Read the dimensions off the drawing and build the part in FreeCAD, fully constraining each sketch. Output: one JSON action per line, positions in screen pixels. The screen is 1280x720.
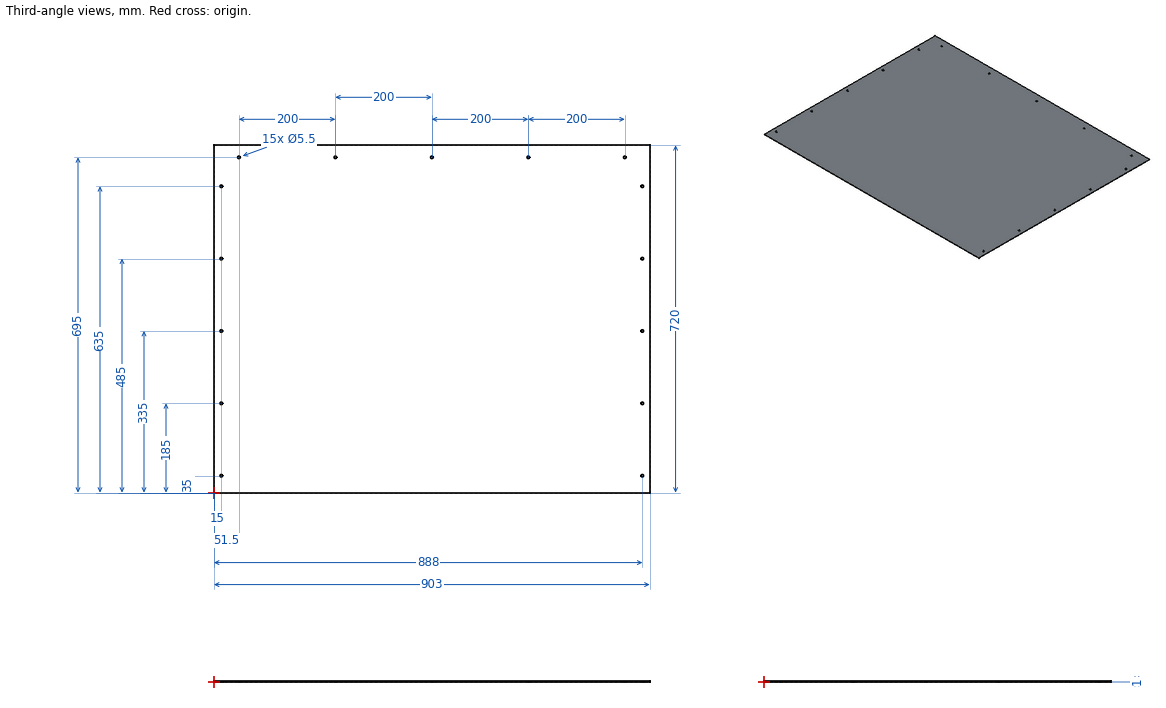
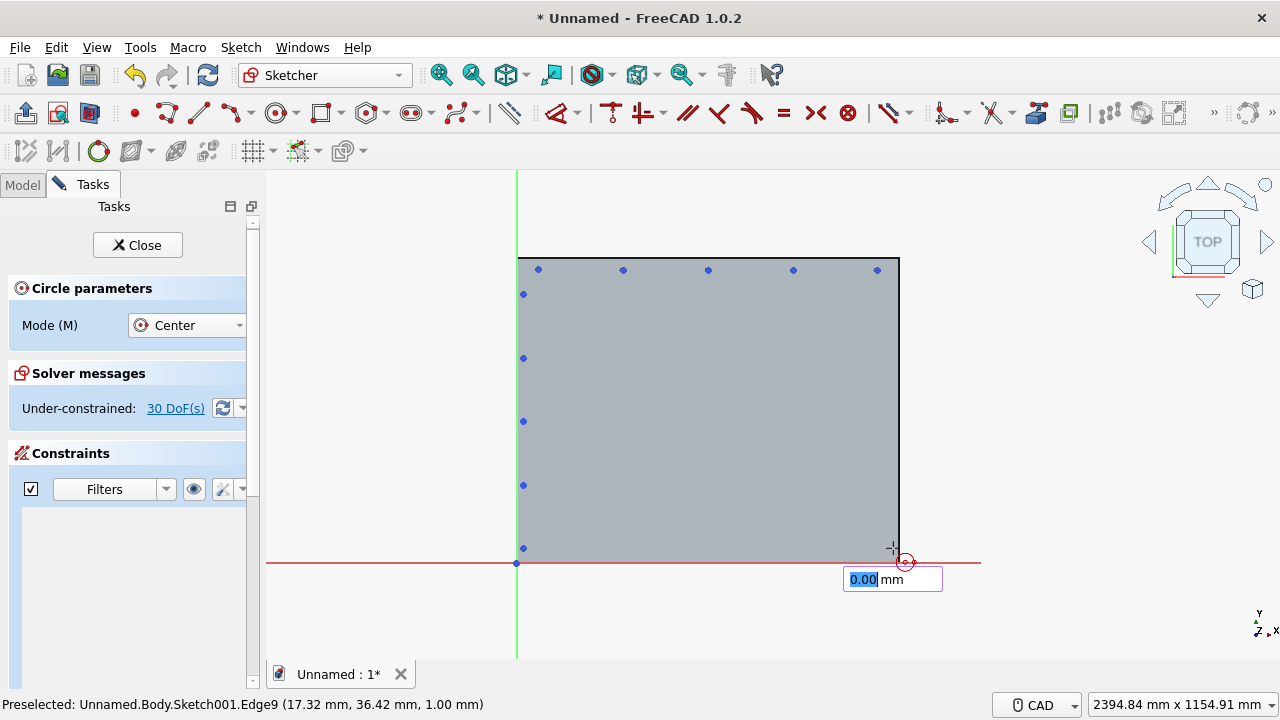
{"action": "scroll", "coordinate": [894, 547], "scroll_direction": "up", "scroll_amount": 14}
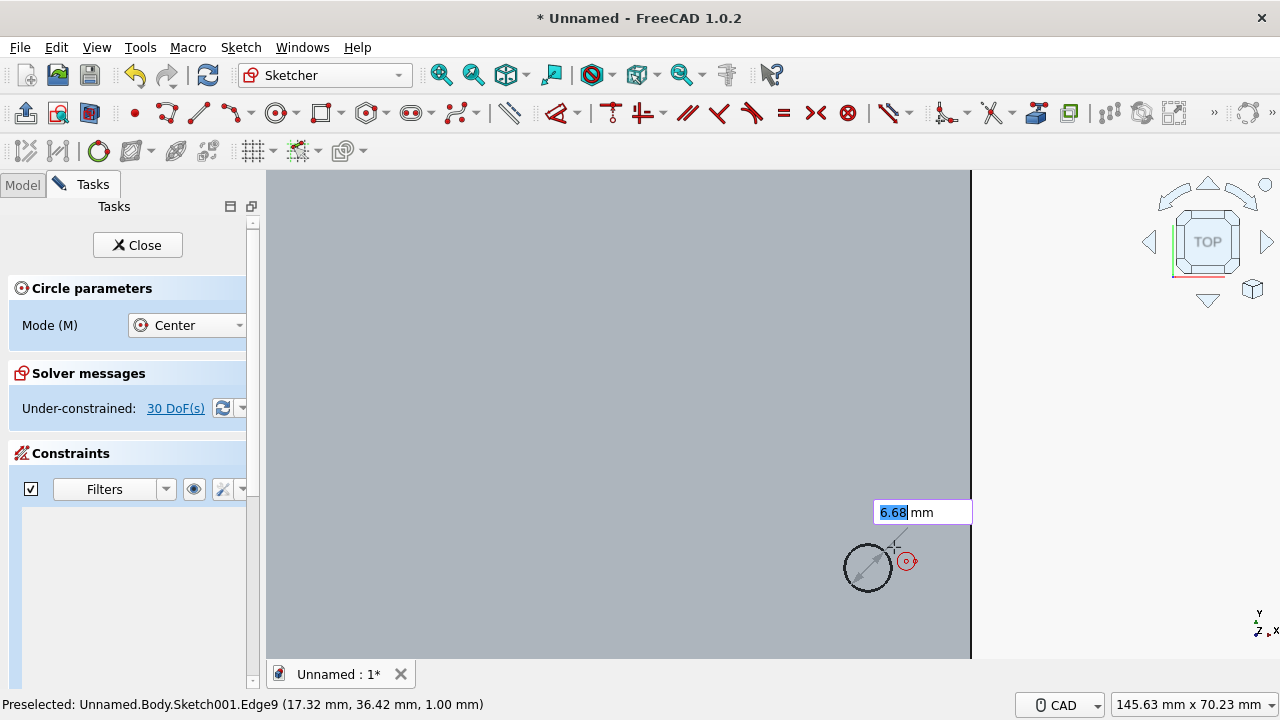
{"action": "left_click", "coordinate": [880, 541]}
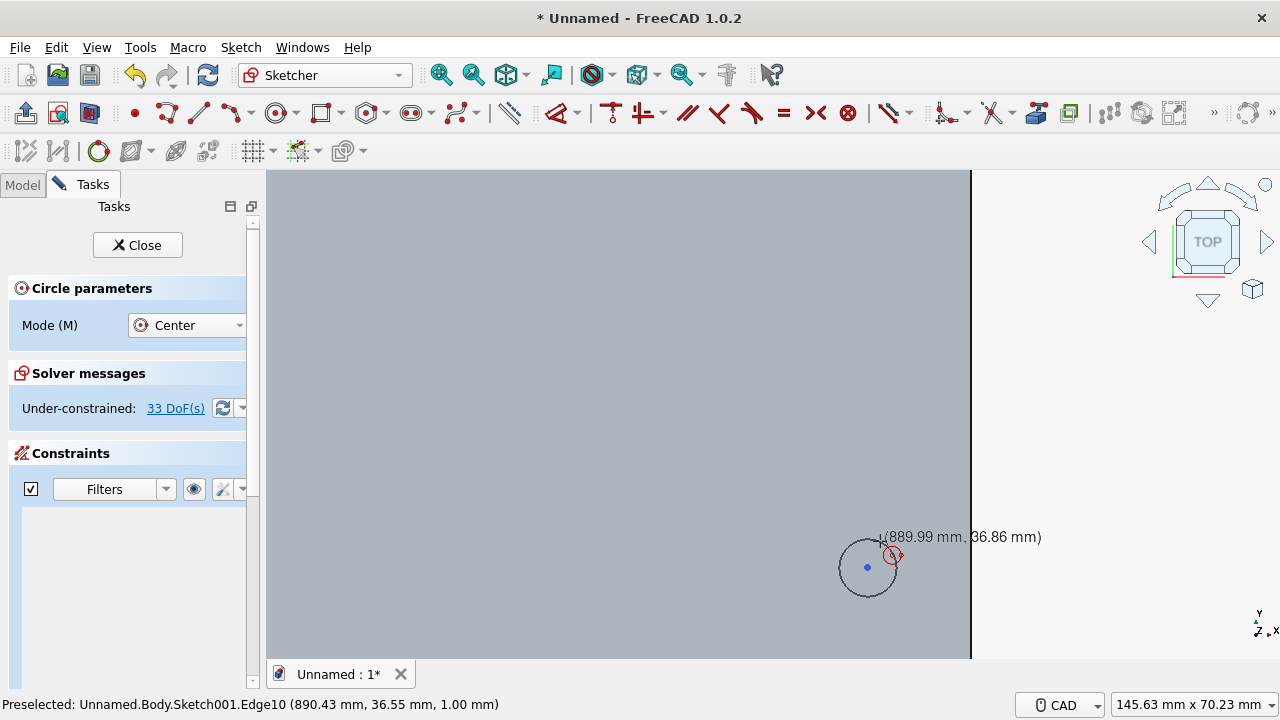
{"action": "scroll", "coordinate": [894, 547], "scroll_direction": "down", "scroll_amount": 14}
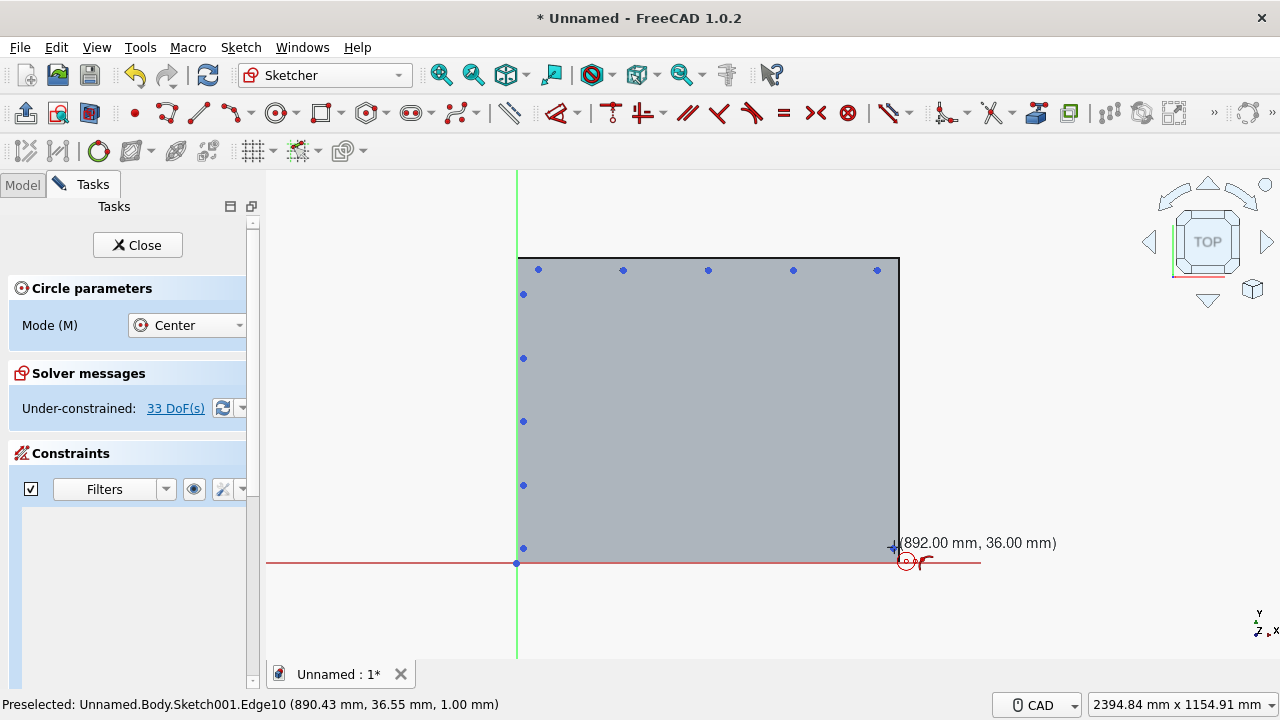
{"action": "scroll", "coordinate": [893, 485], "scroll_direction": "up", "scroll_amount": 15}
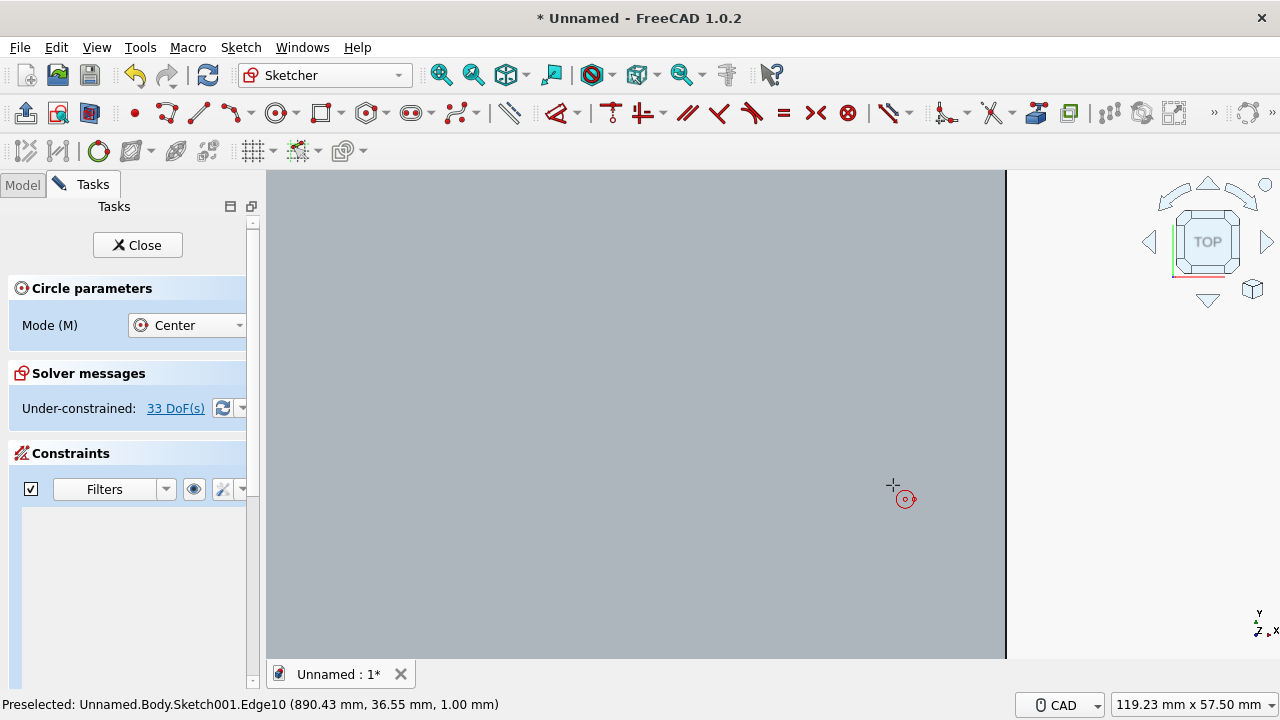
{"action": "scroll", "coordinate": [893, 485], "scroll_direction": "down", "scroll_amount": 15}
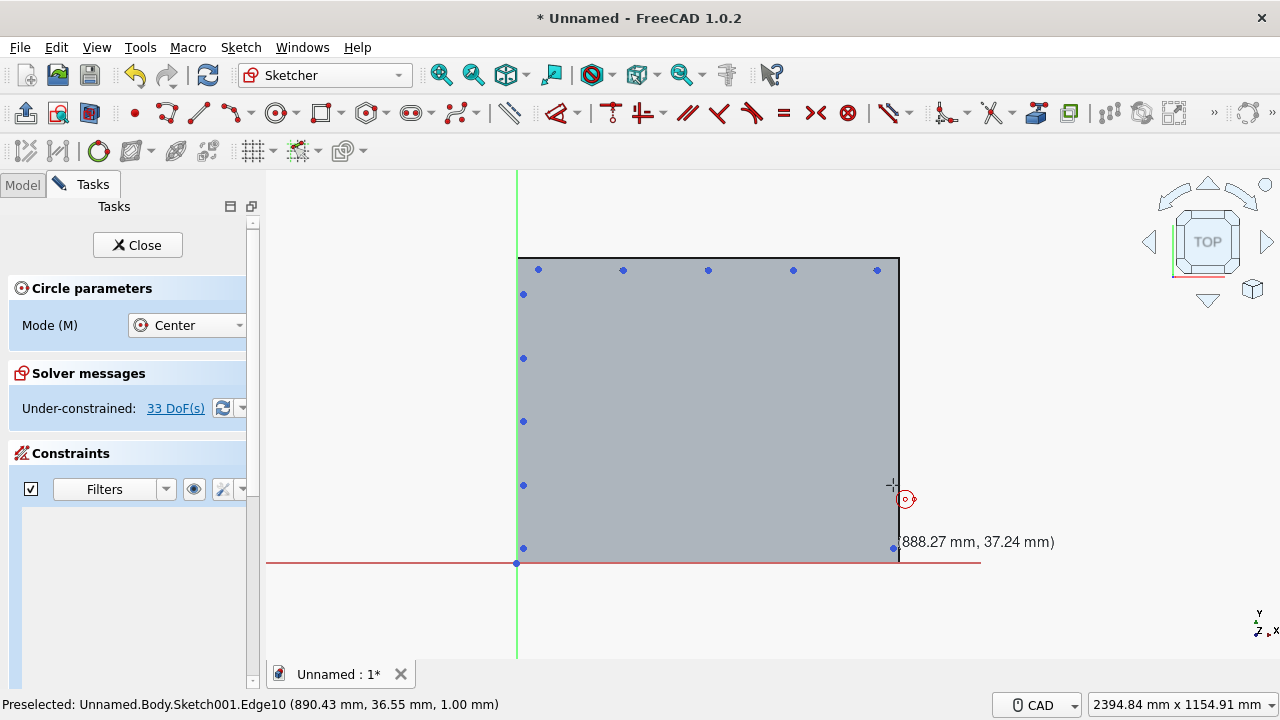
{"action": "left_click", "coordinate": [893, 485]}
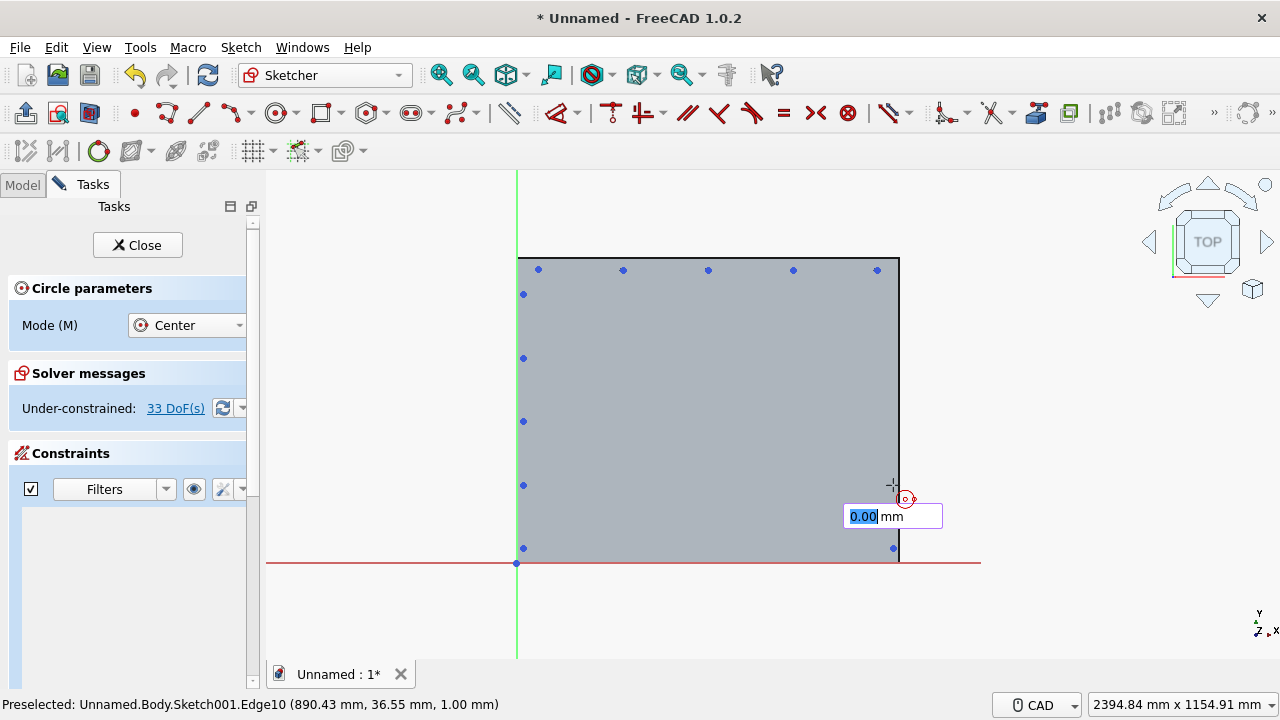
{"action": "scroll", "coordinate": [894, 484], "scroll_direction": "up", "scroll_amount": 14}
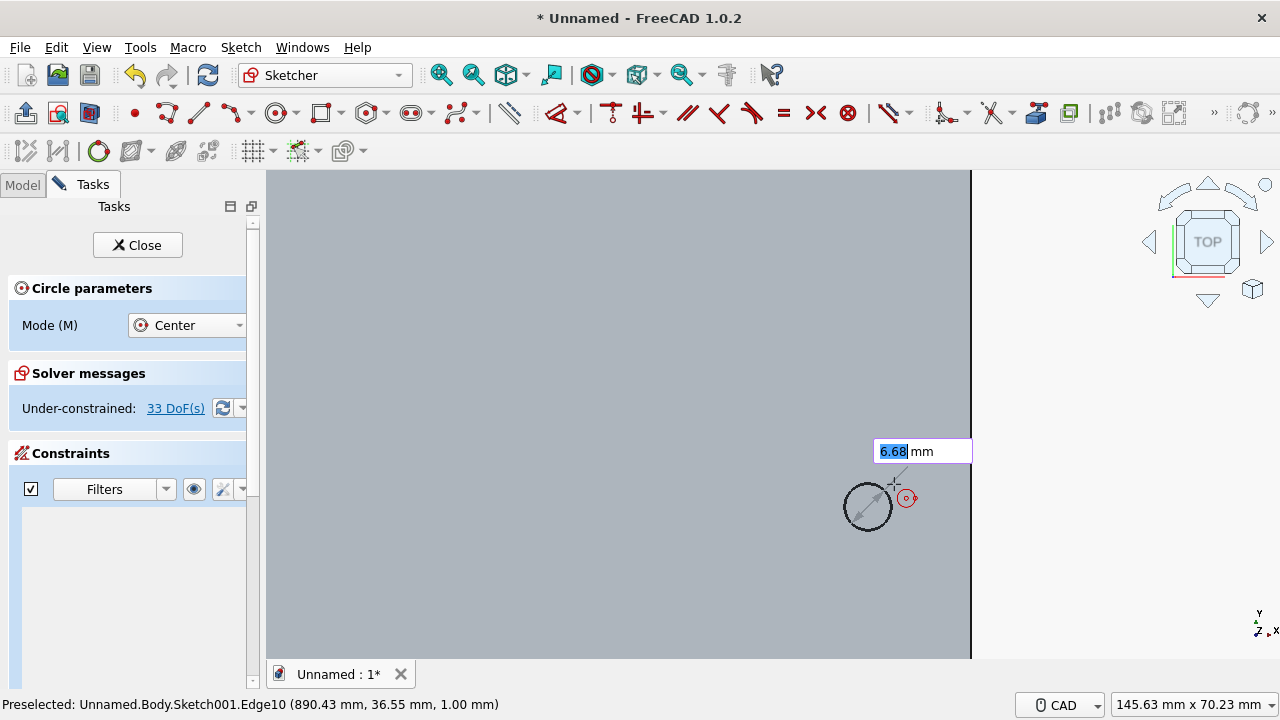
{"action": "left_click", "coordinate": [880, 472]}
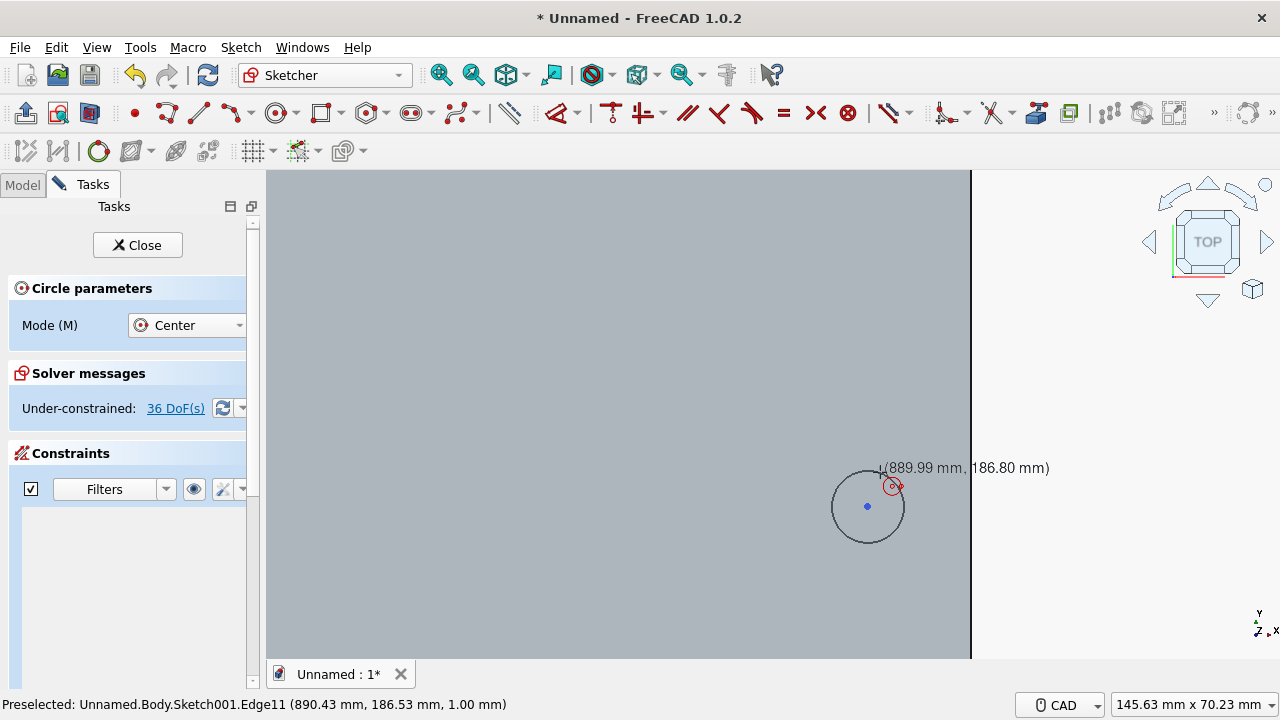
{"action": "scroll", "coordinate": [894, 484], "scroll_direction": "down", "scroll_amount": 14}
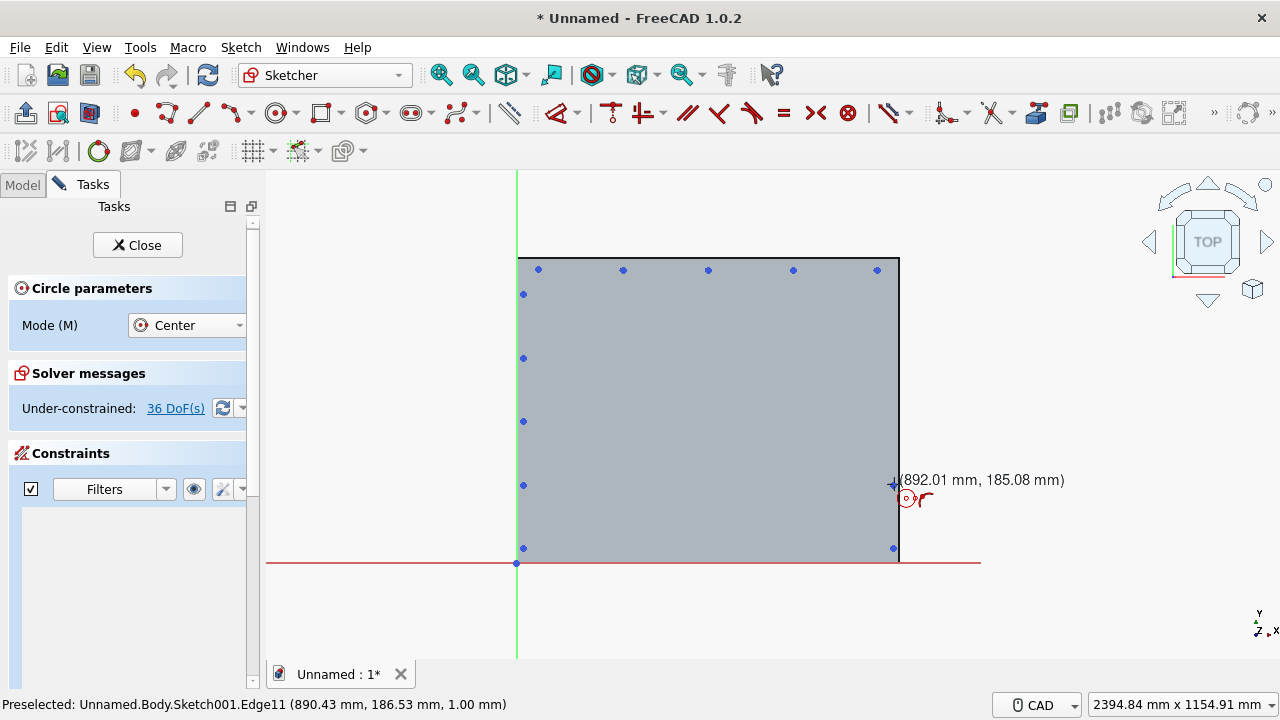
{"action": "scroll", "coordinate": [893, 421], "scroll_direction": "up", "scroll_amount": 15}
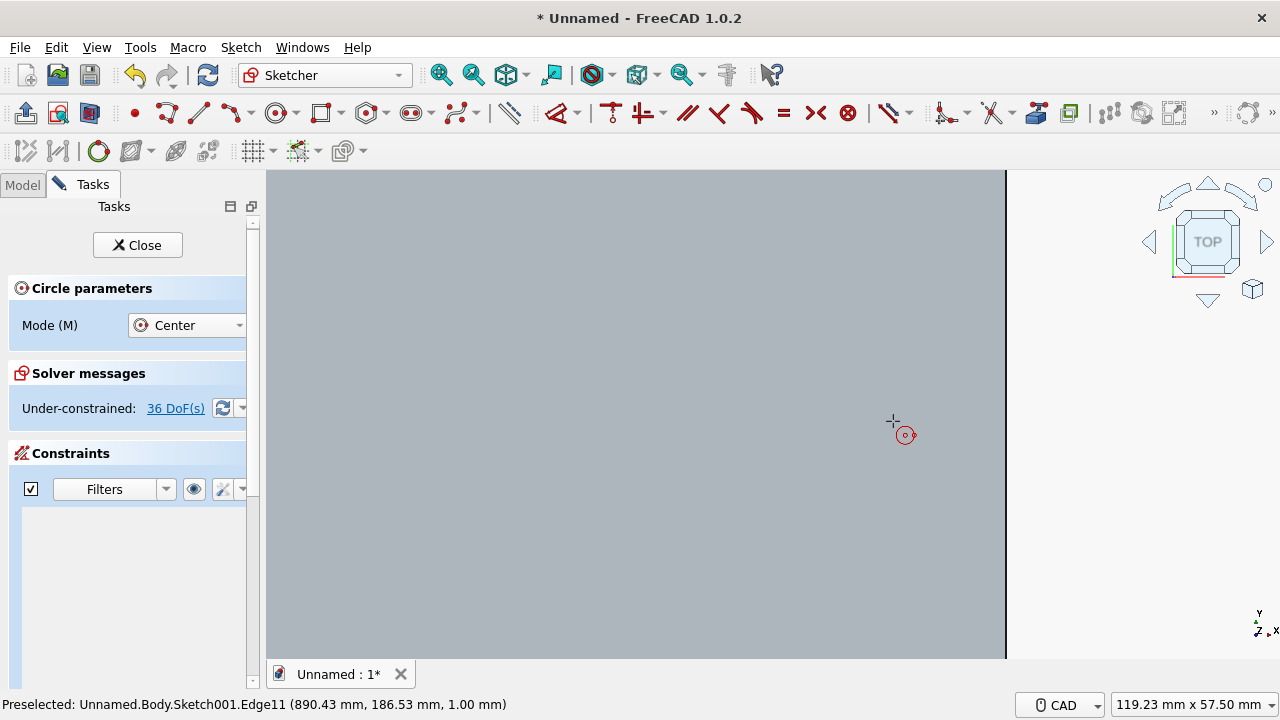
{"action": "scroll", "coordinate": [893, 421], "scroll_direction": "down", "scroll_amount": 15}